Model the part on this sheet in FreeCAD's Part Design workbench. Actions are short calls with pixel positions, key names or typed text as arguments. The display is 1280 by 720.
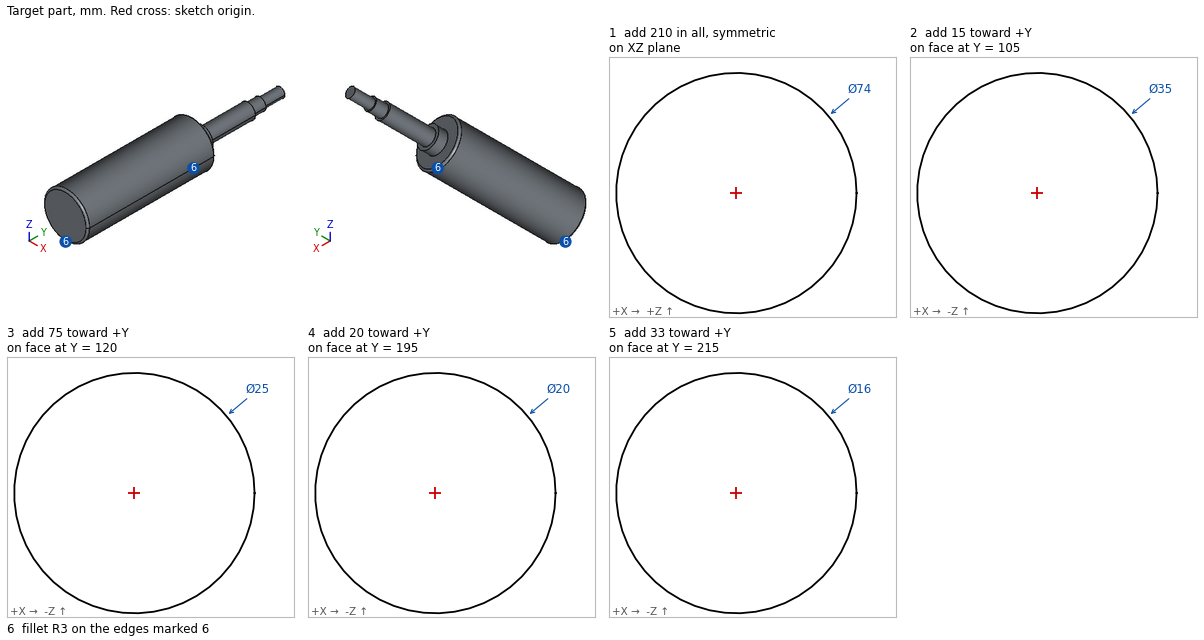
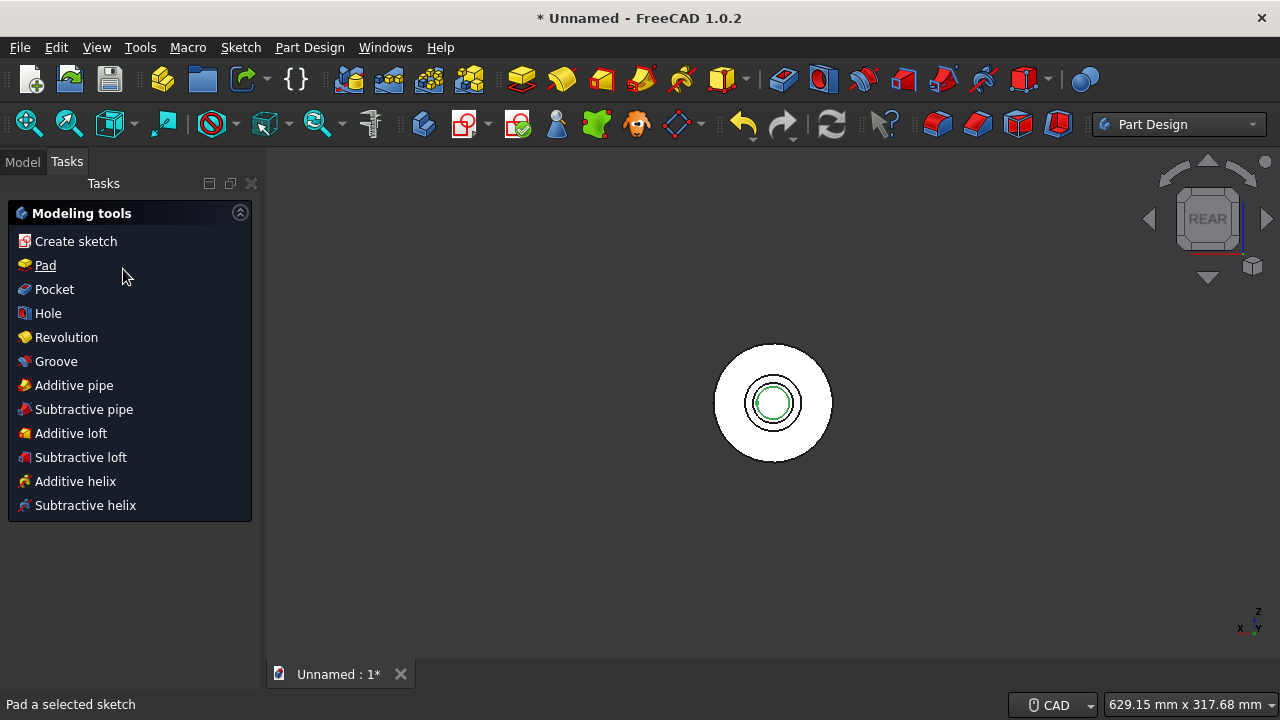
click(522, 80)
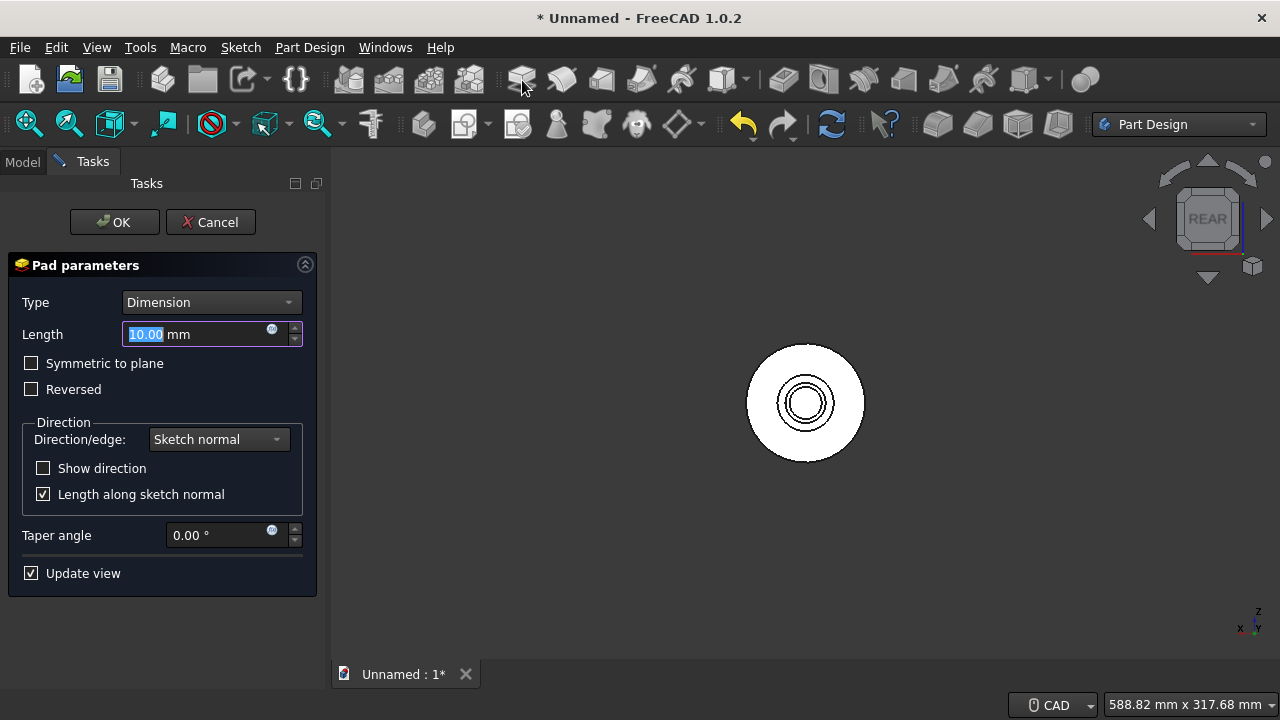
text(20)
key(Tab)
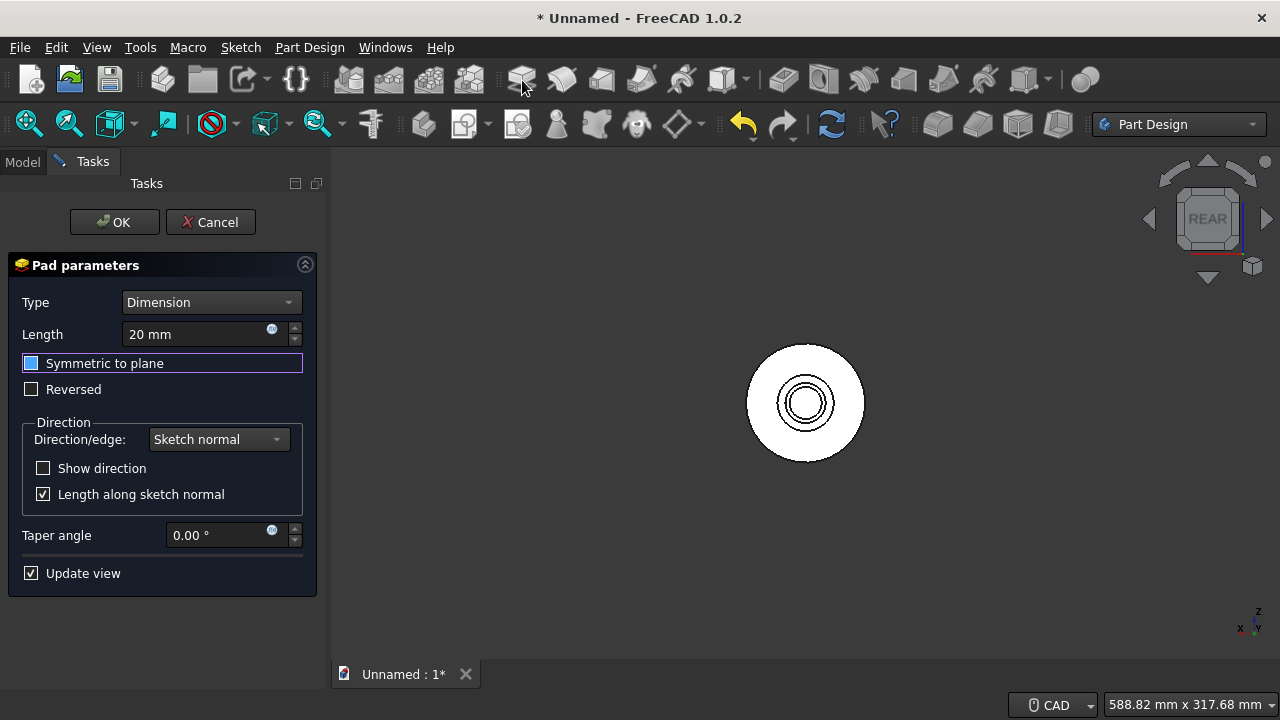
click(115, 222)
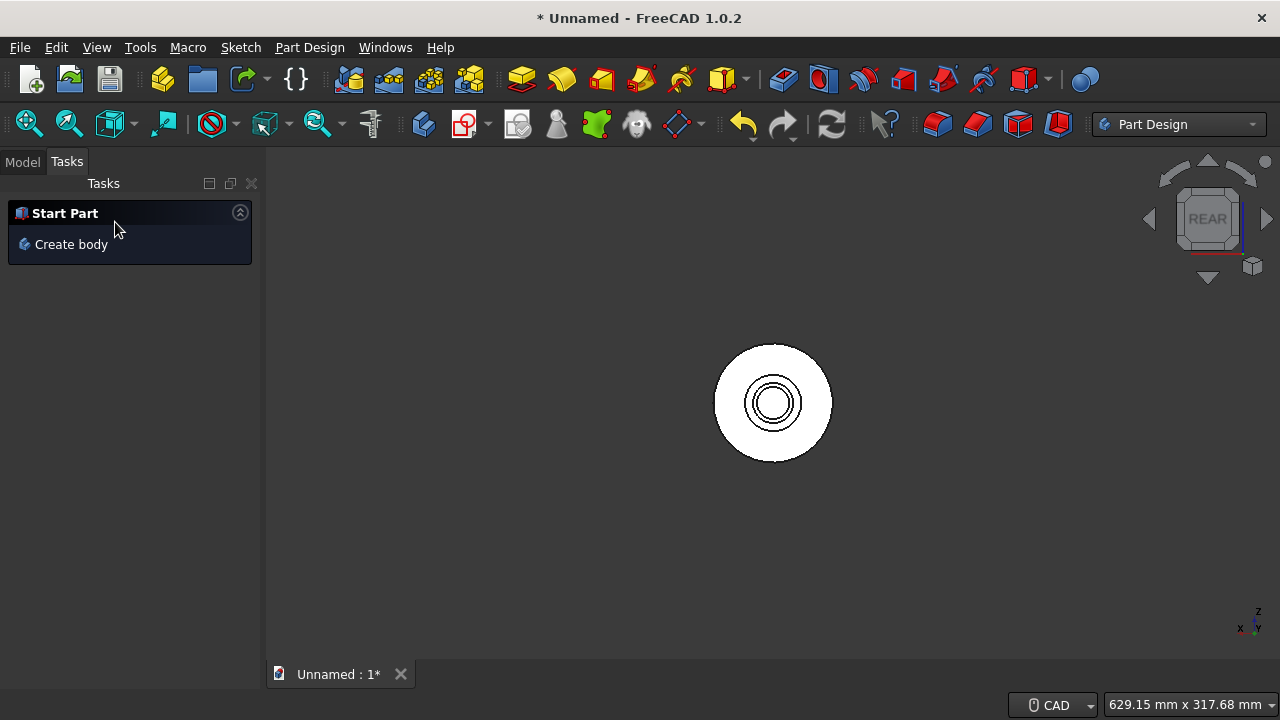
click(30, 124)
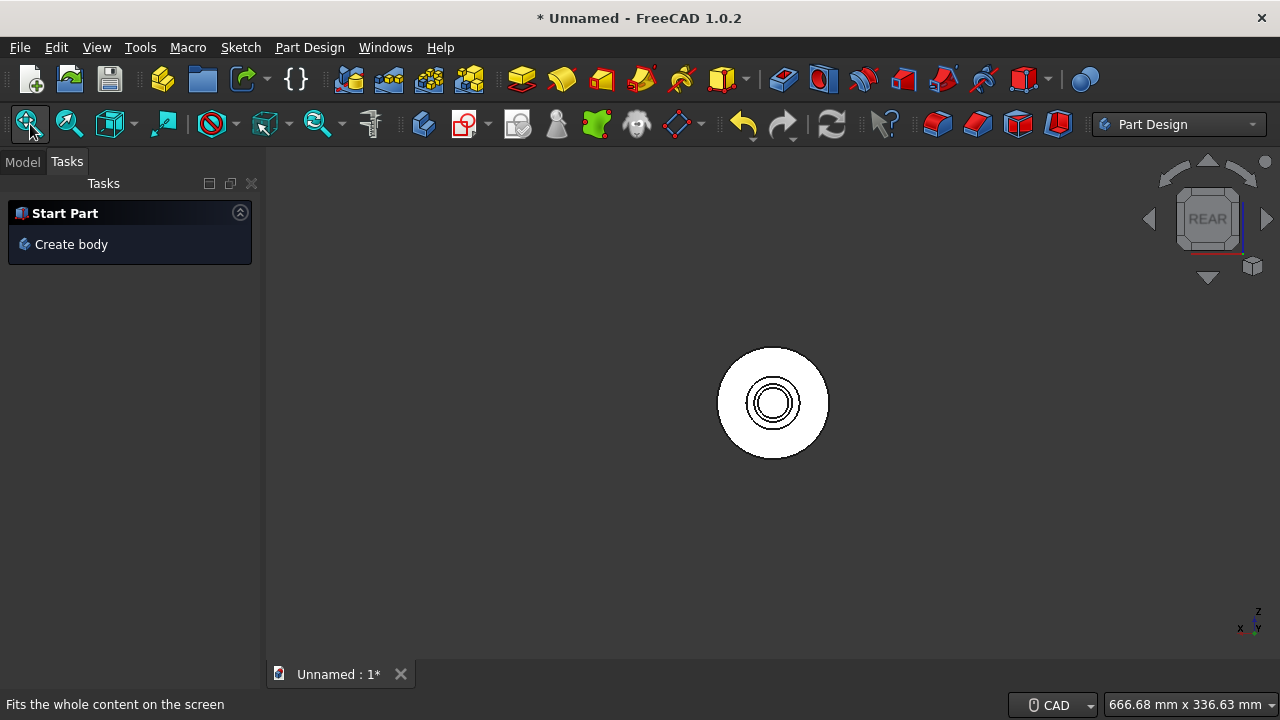
click(773, 402)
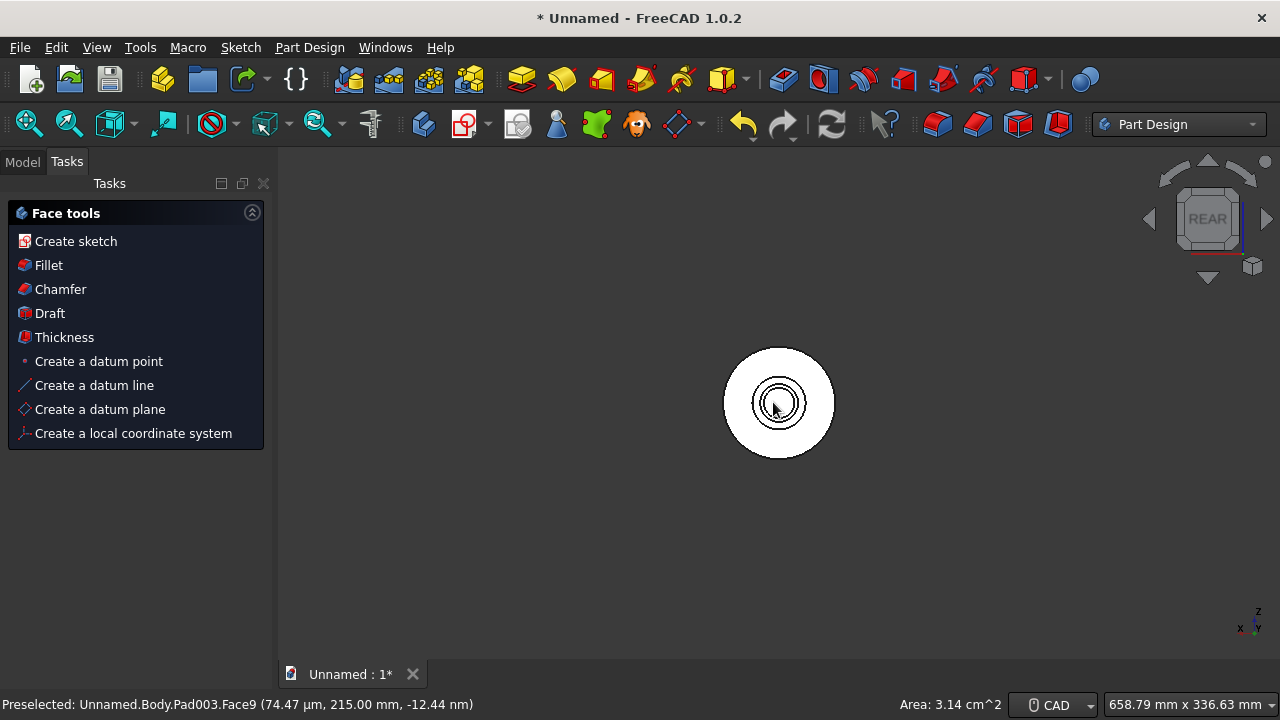
click(464, 124)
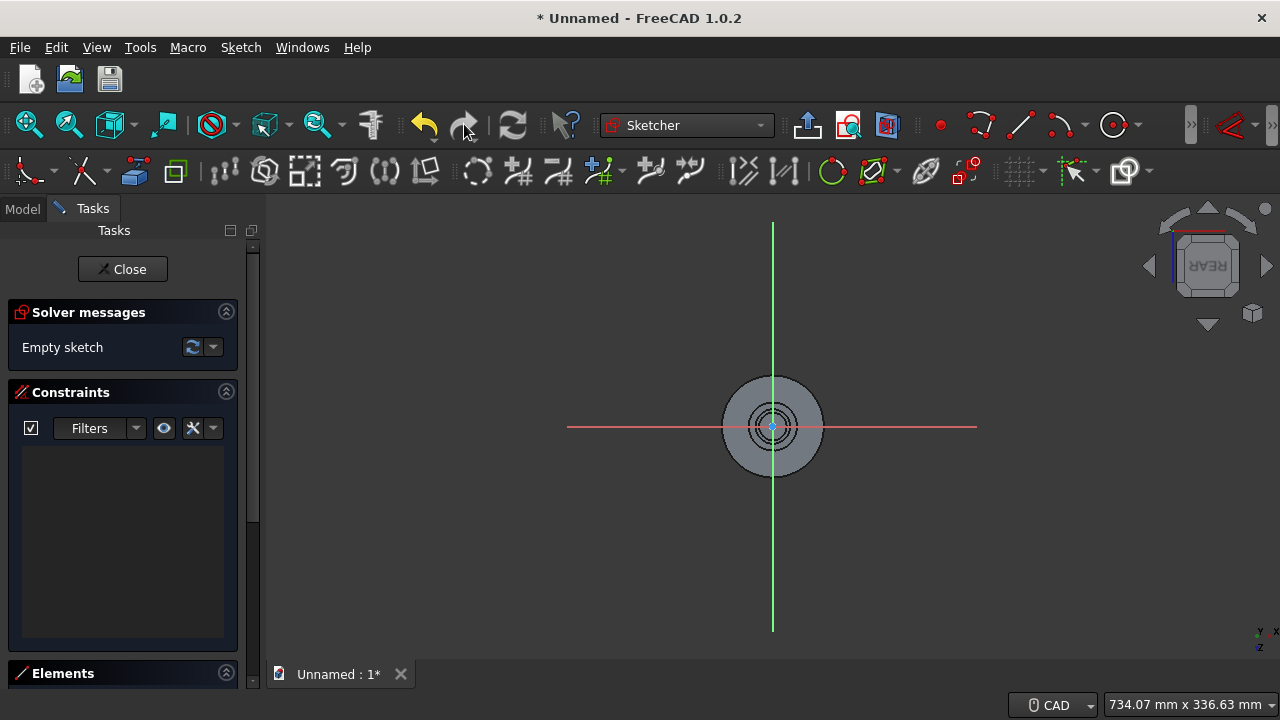
scroll(778, 426, up, 13)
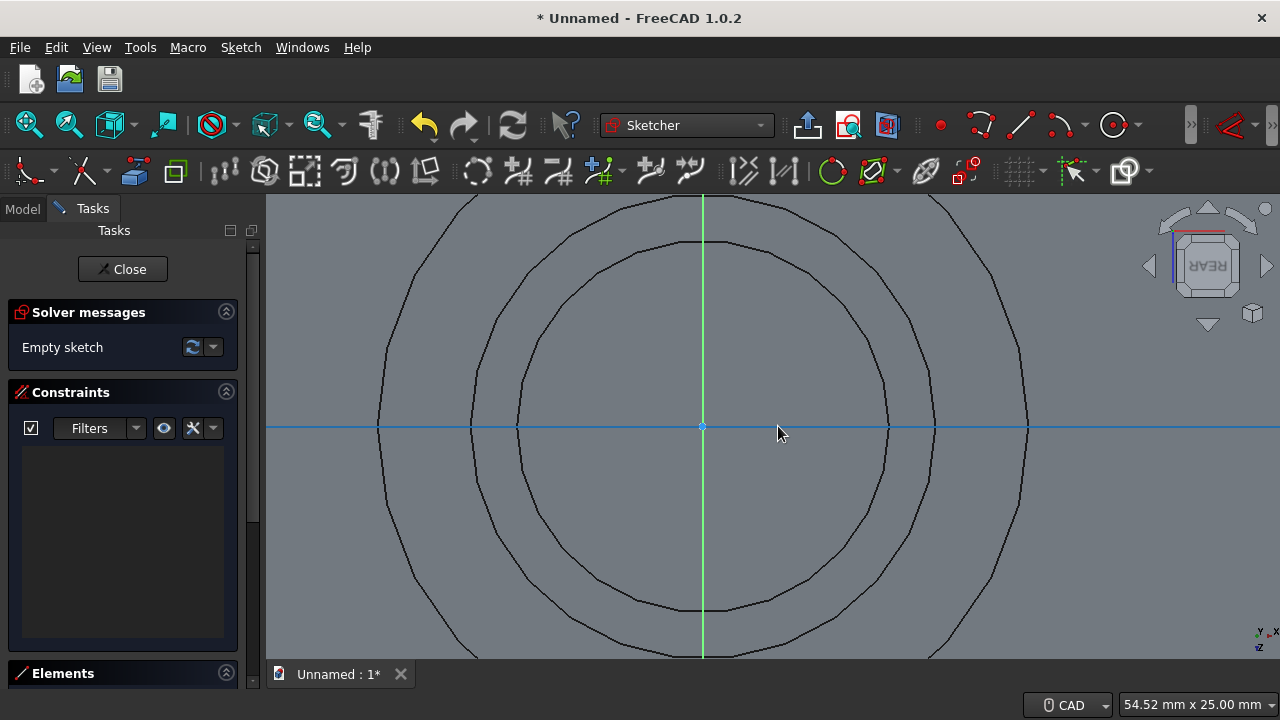
click(1114, 126)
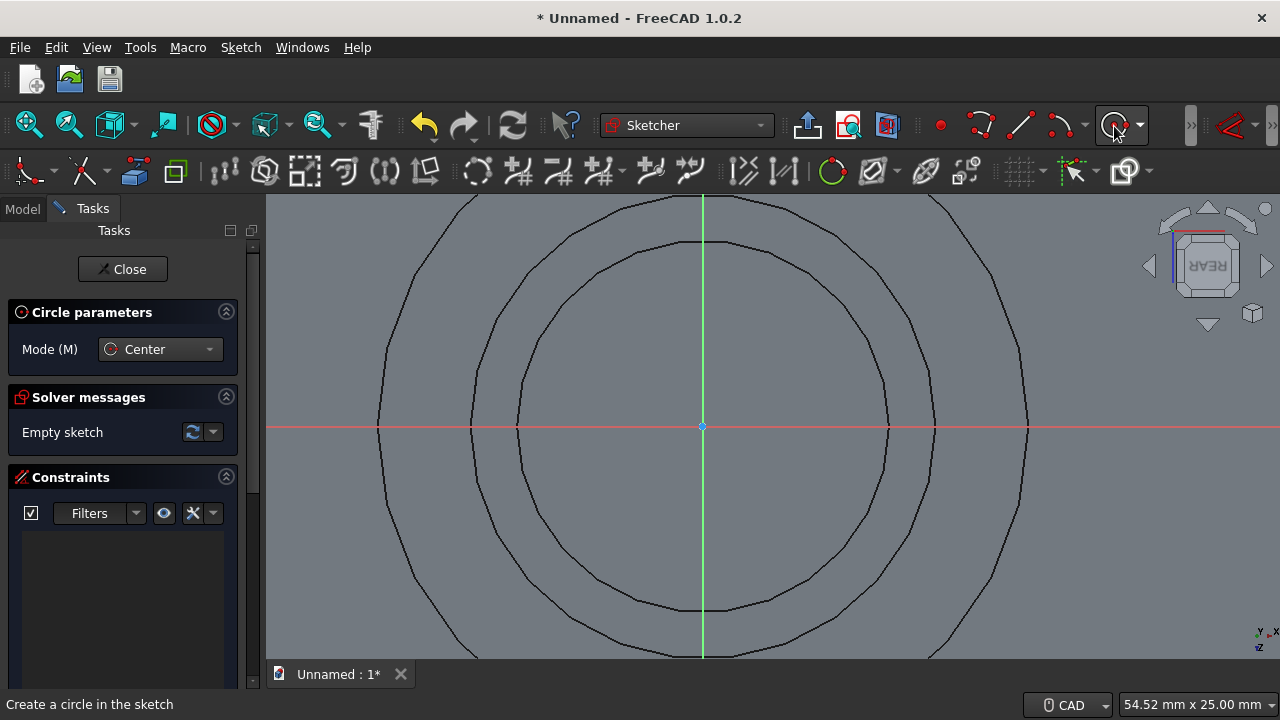
click(703, 426)
move(808, 321)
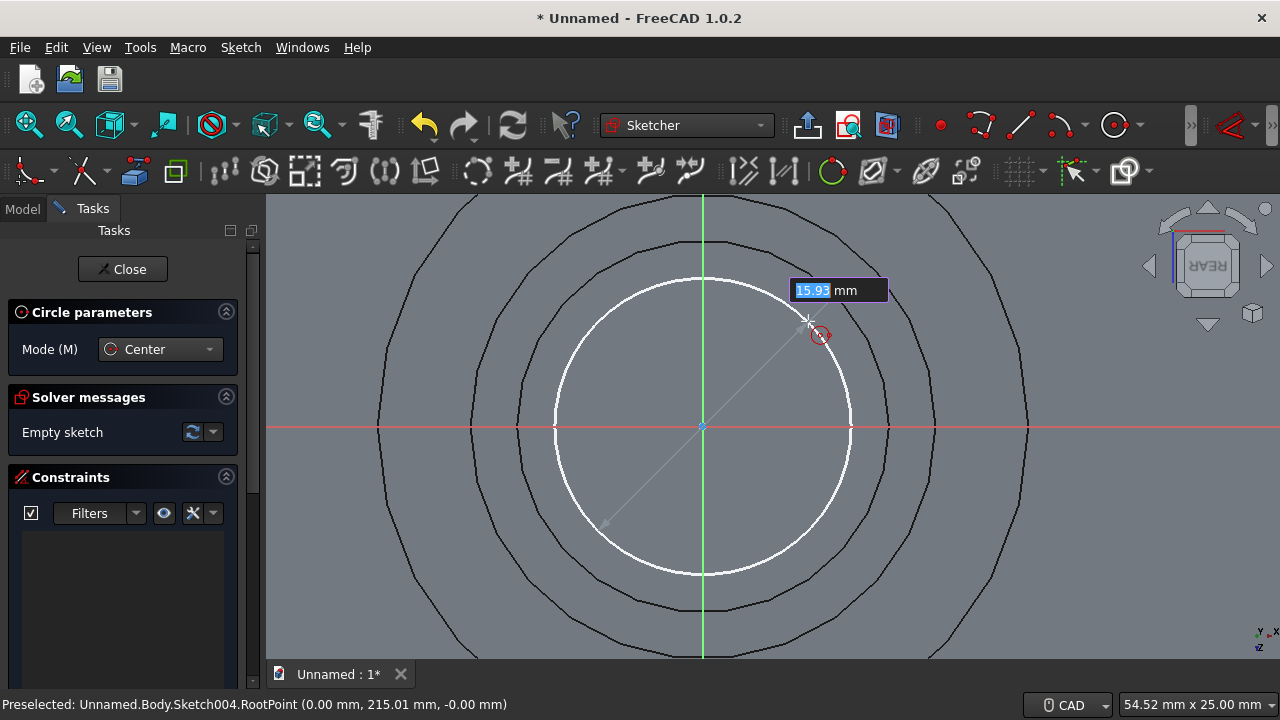
text(16)
key(Return)
key(Escape)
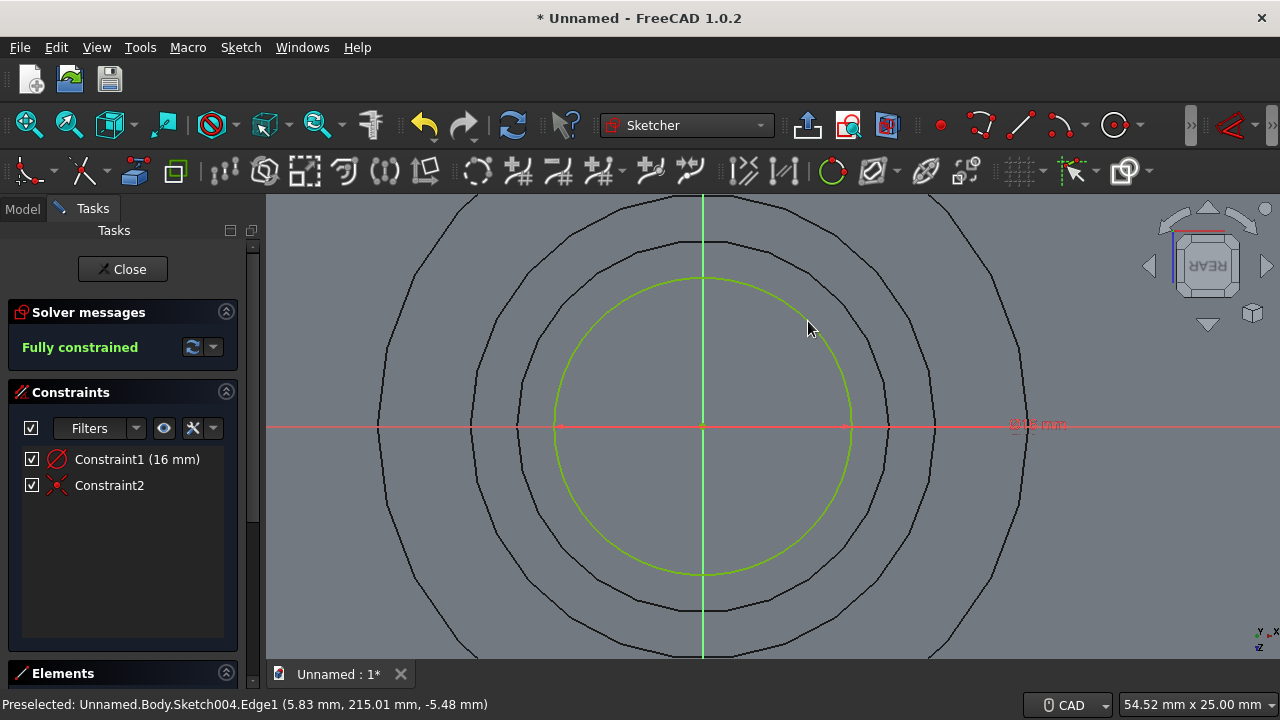
click(123, 269)